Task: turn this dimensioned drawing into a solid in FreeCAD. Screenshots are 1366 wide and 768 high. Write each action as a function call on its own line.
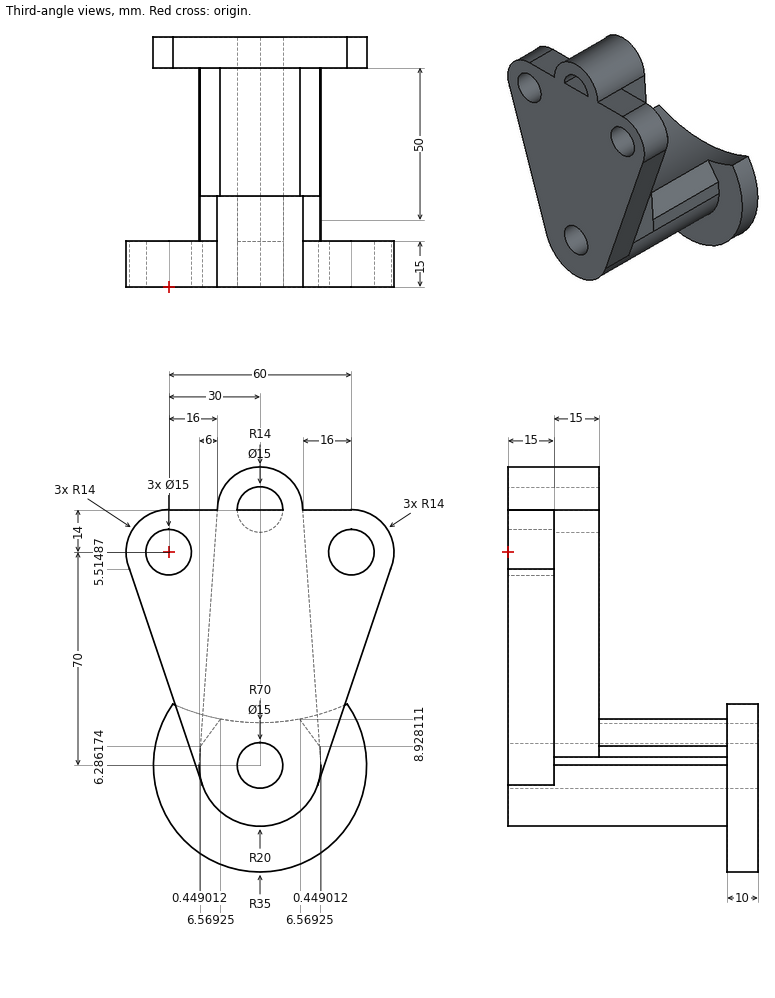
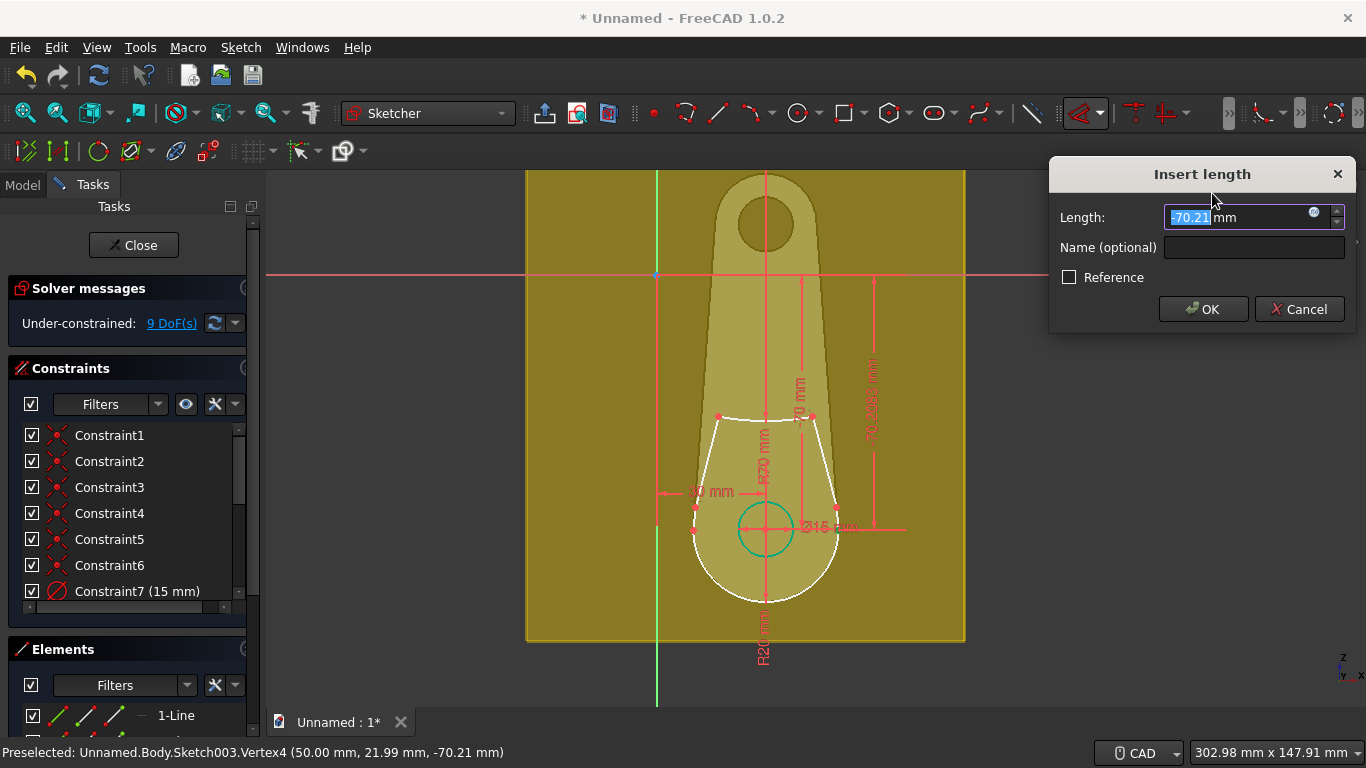
text(-70)
key(Return)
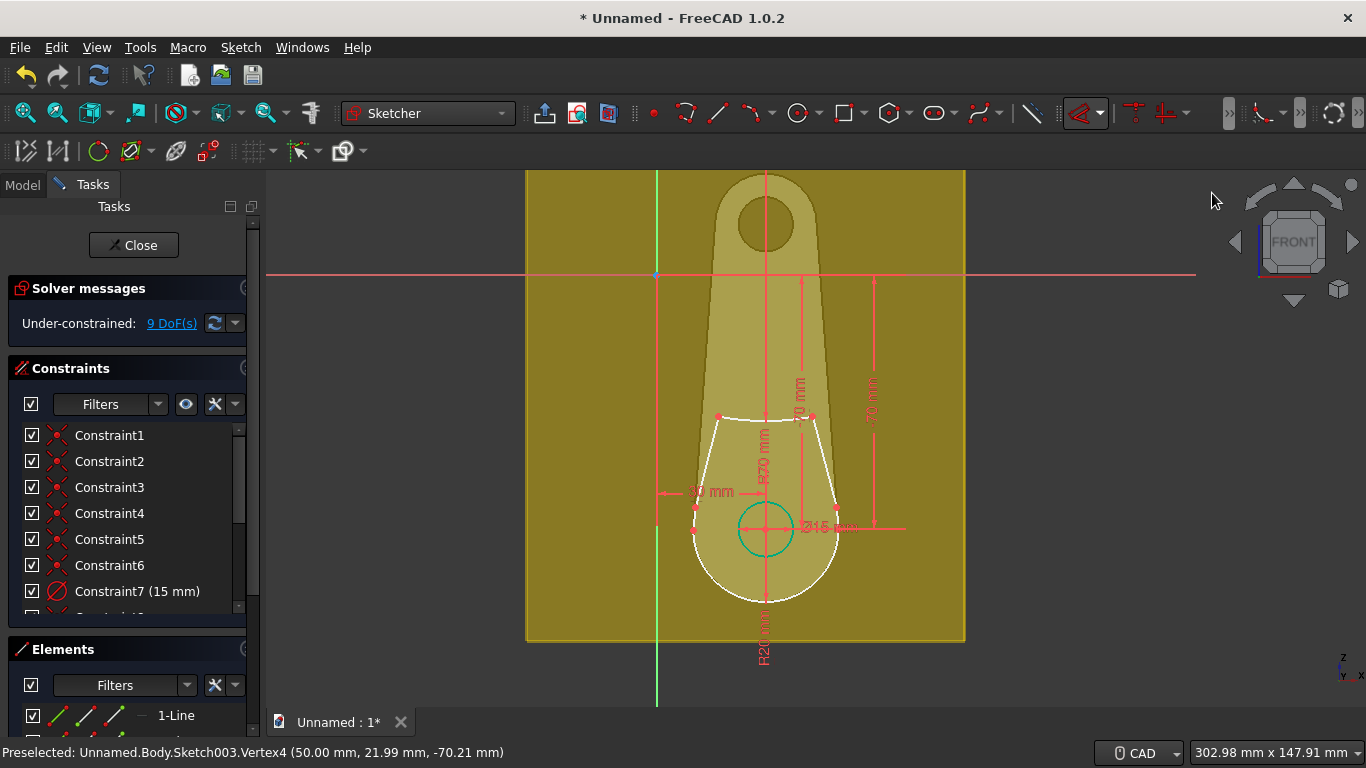
click(693, 530)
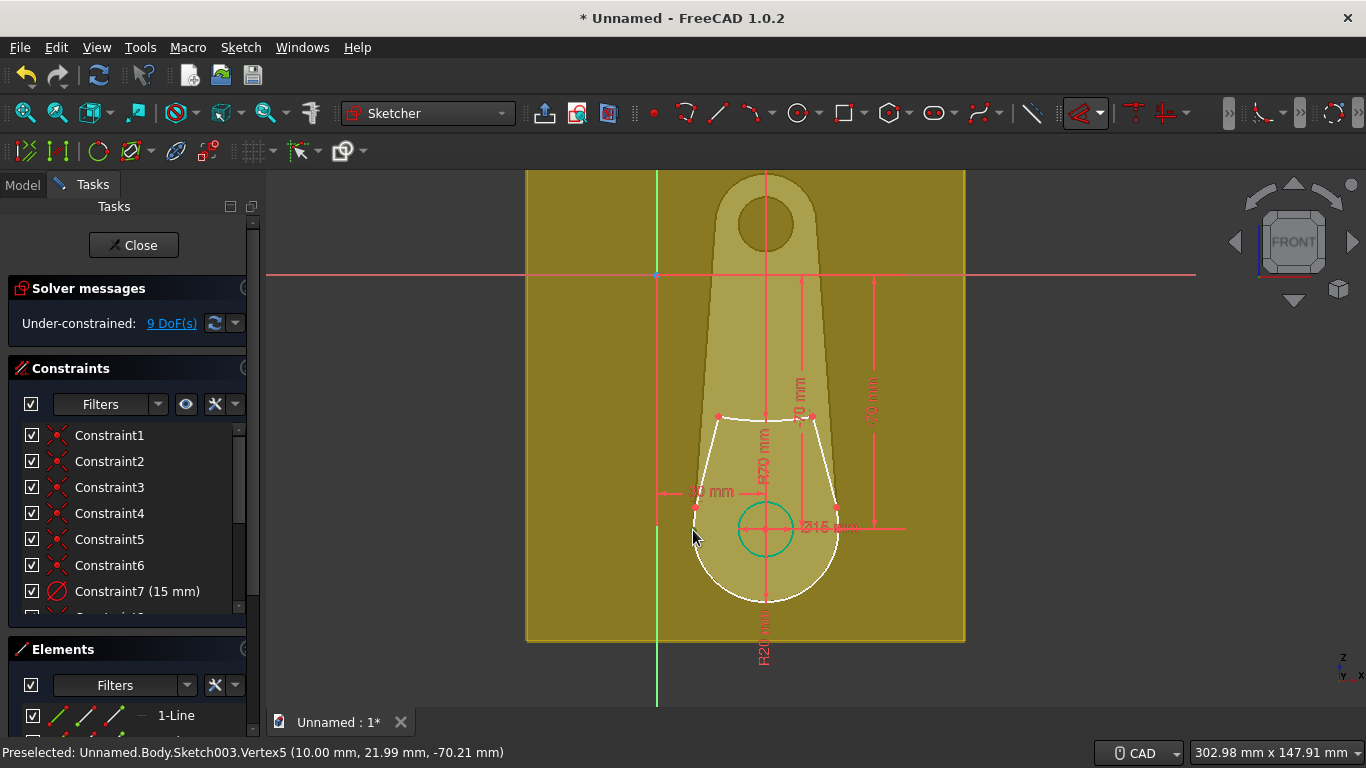
click(1102, 114)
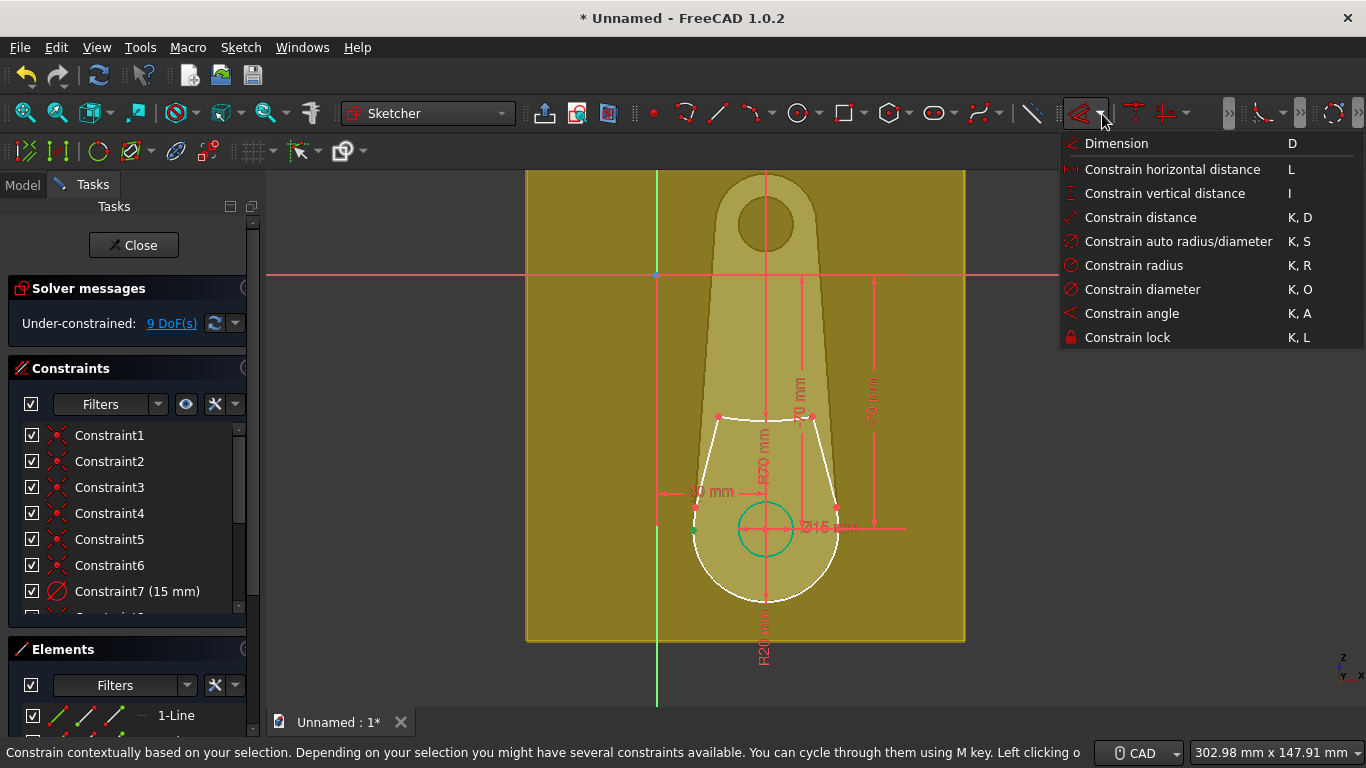
click(1212, 193)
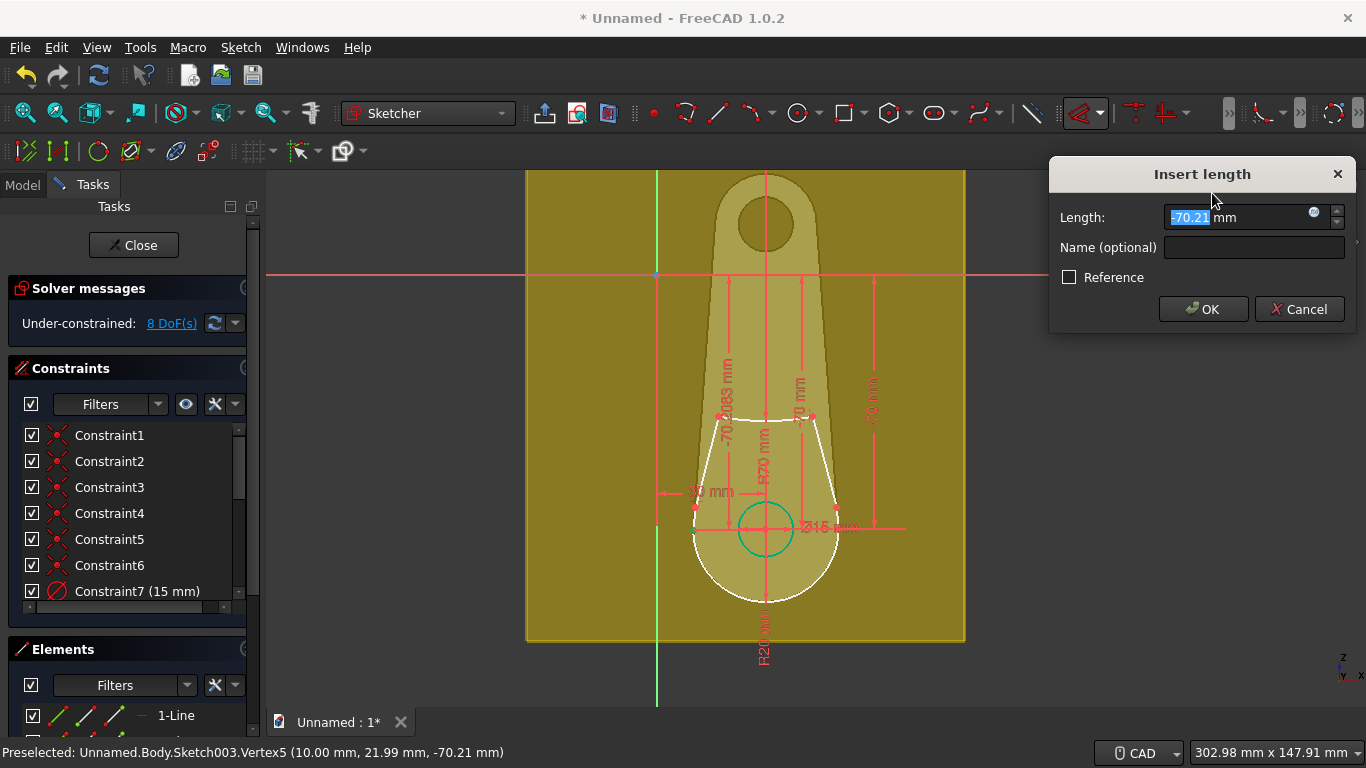
text(-70)
key(Return)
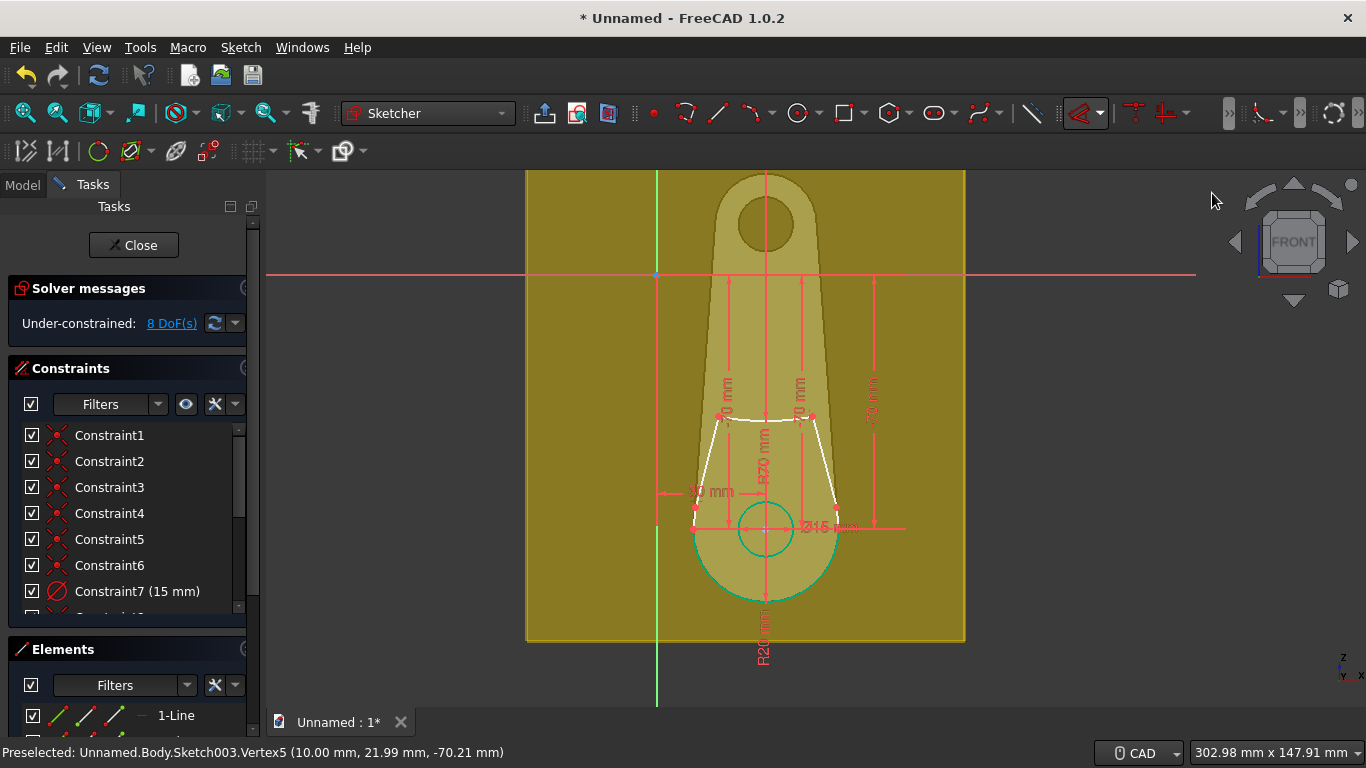
scroll(747, 679, down, 1)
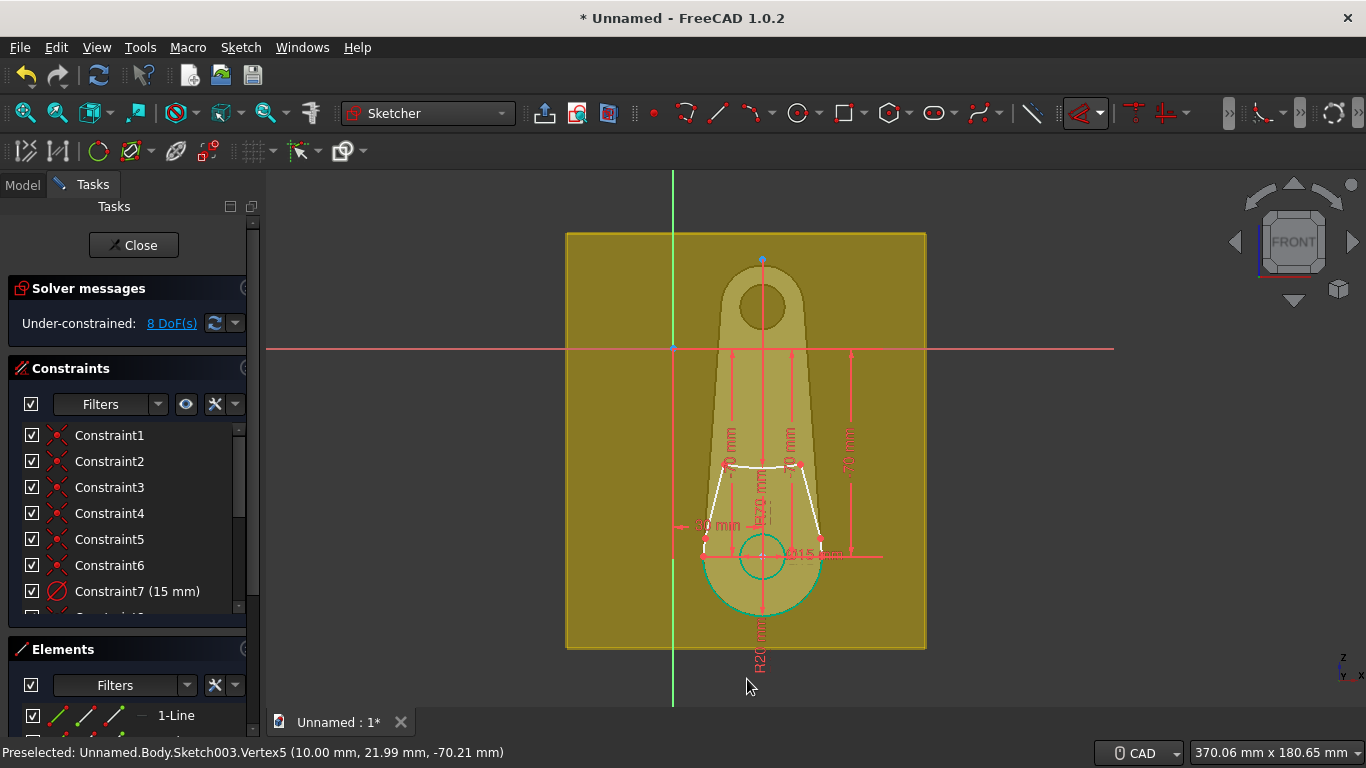
click(763, 260)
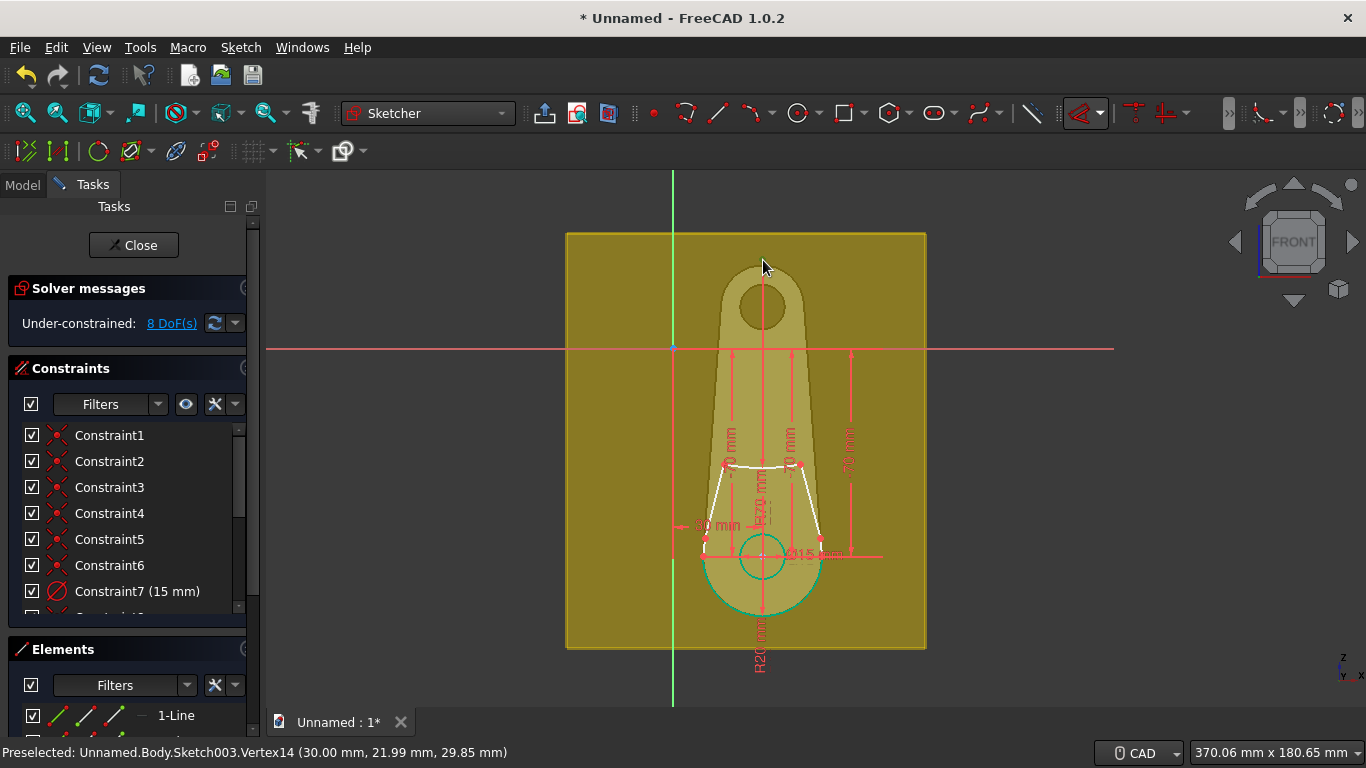
key(l)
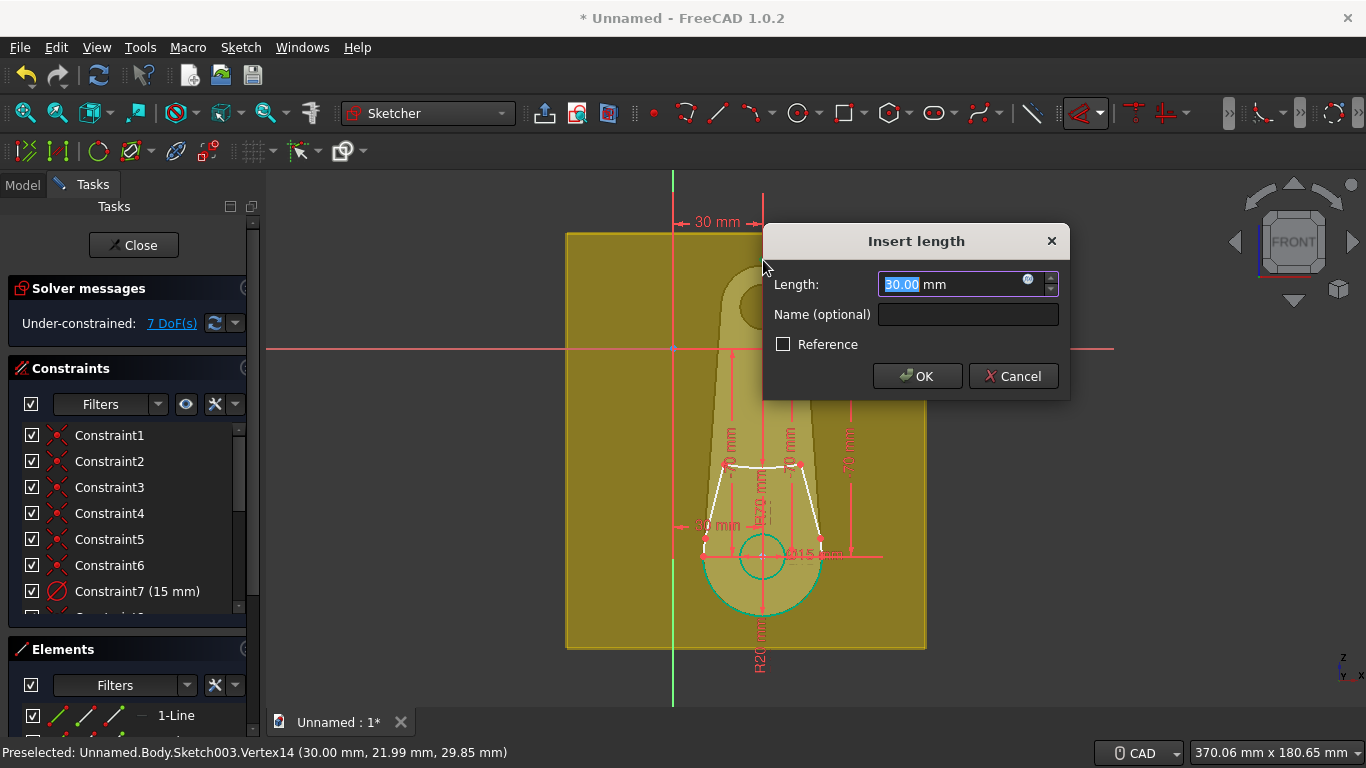
text(30)
key(Return)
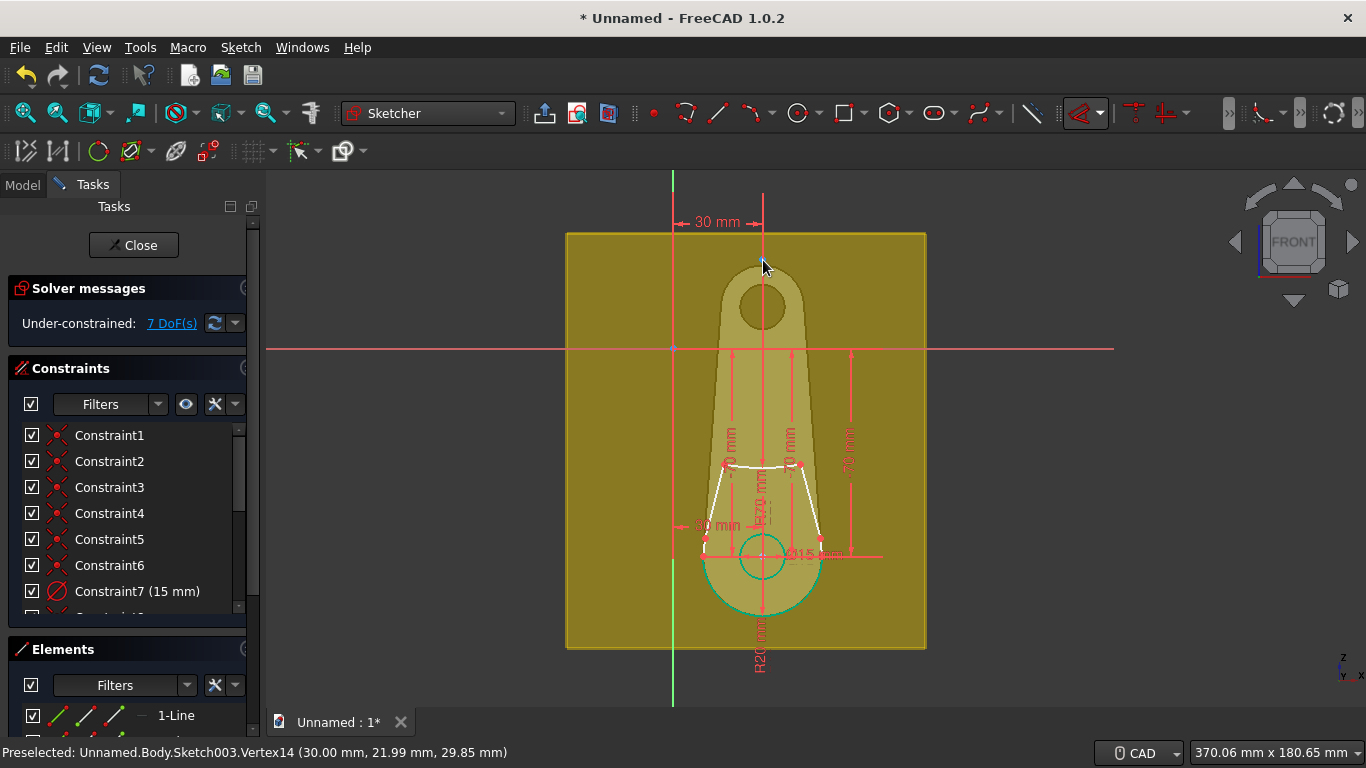
click(763, 260)